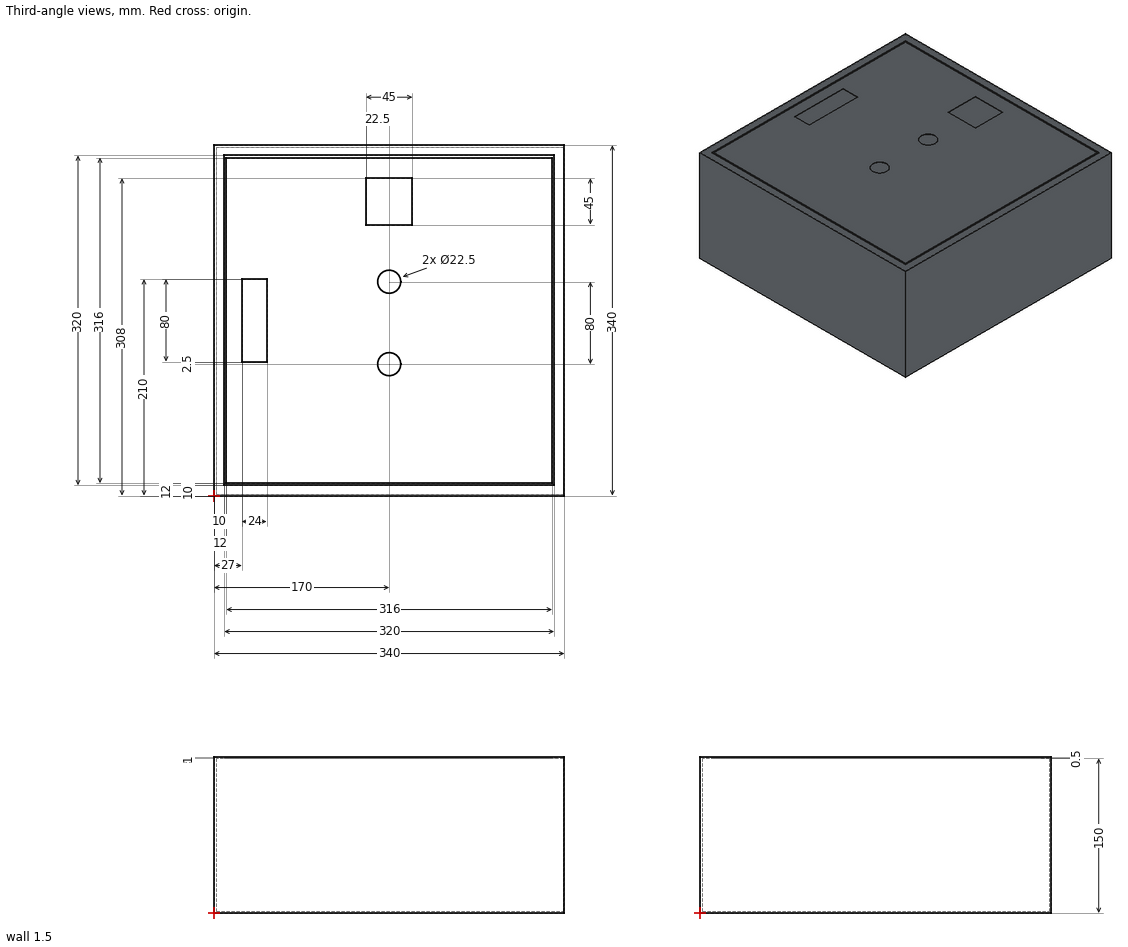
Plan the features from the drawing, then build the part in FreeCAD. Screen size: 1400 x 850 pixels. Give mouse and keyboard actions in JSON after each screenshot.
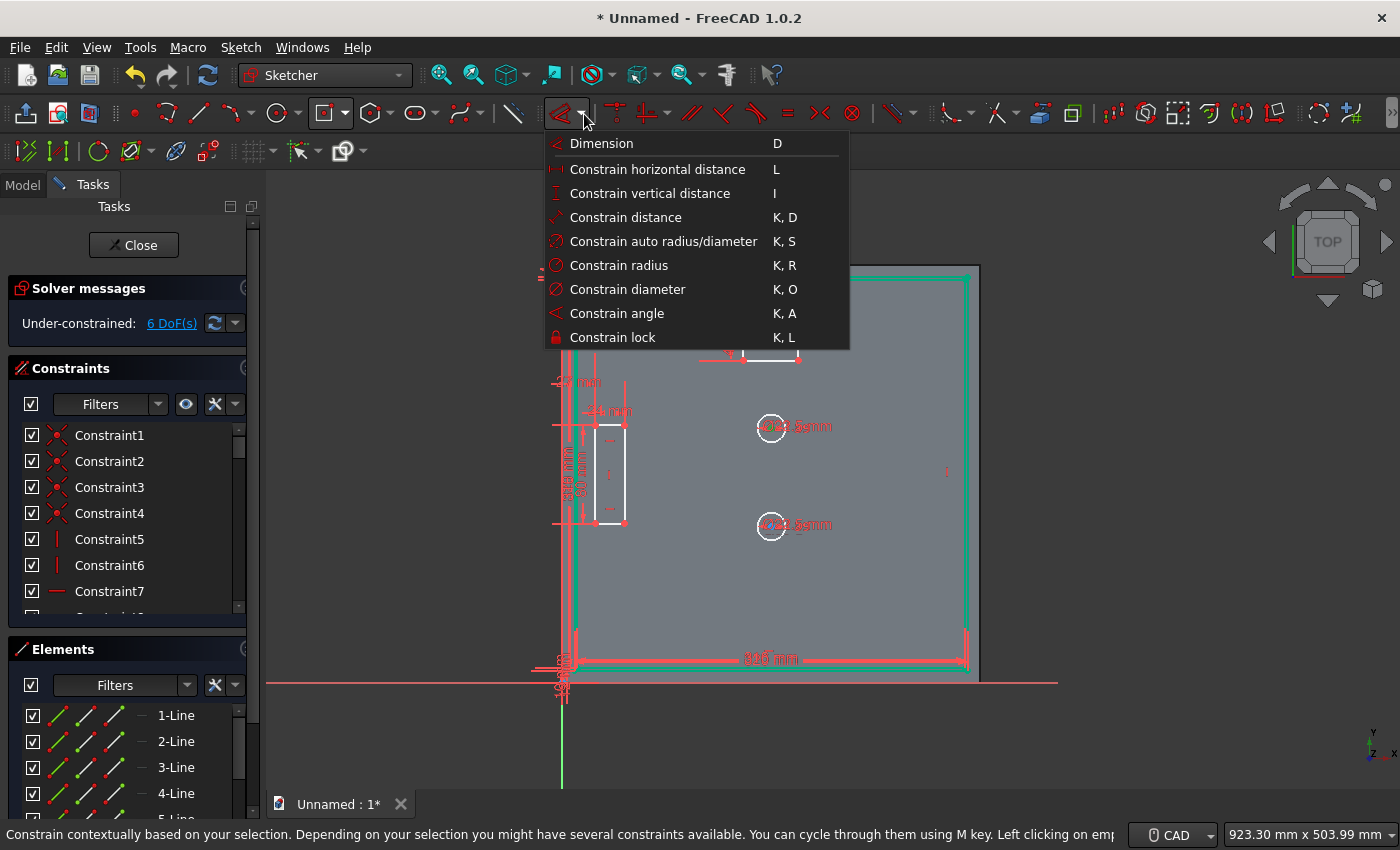
{"action": "left_click", "coordinate": [697, 169]}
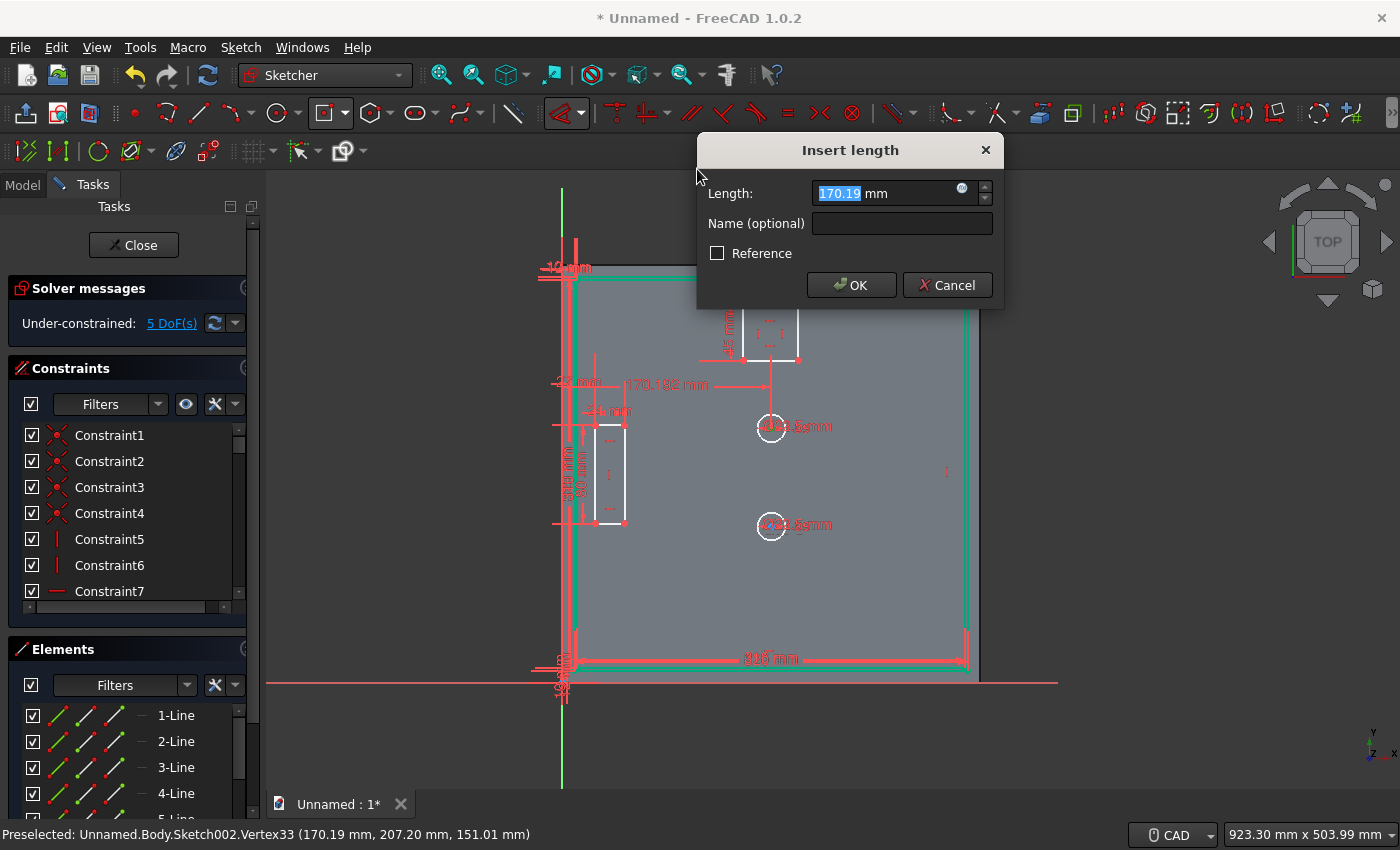
{"action": "type", "text": "170"}
{"action": "key", "text": "Return"}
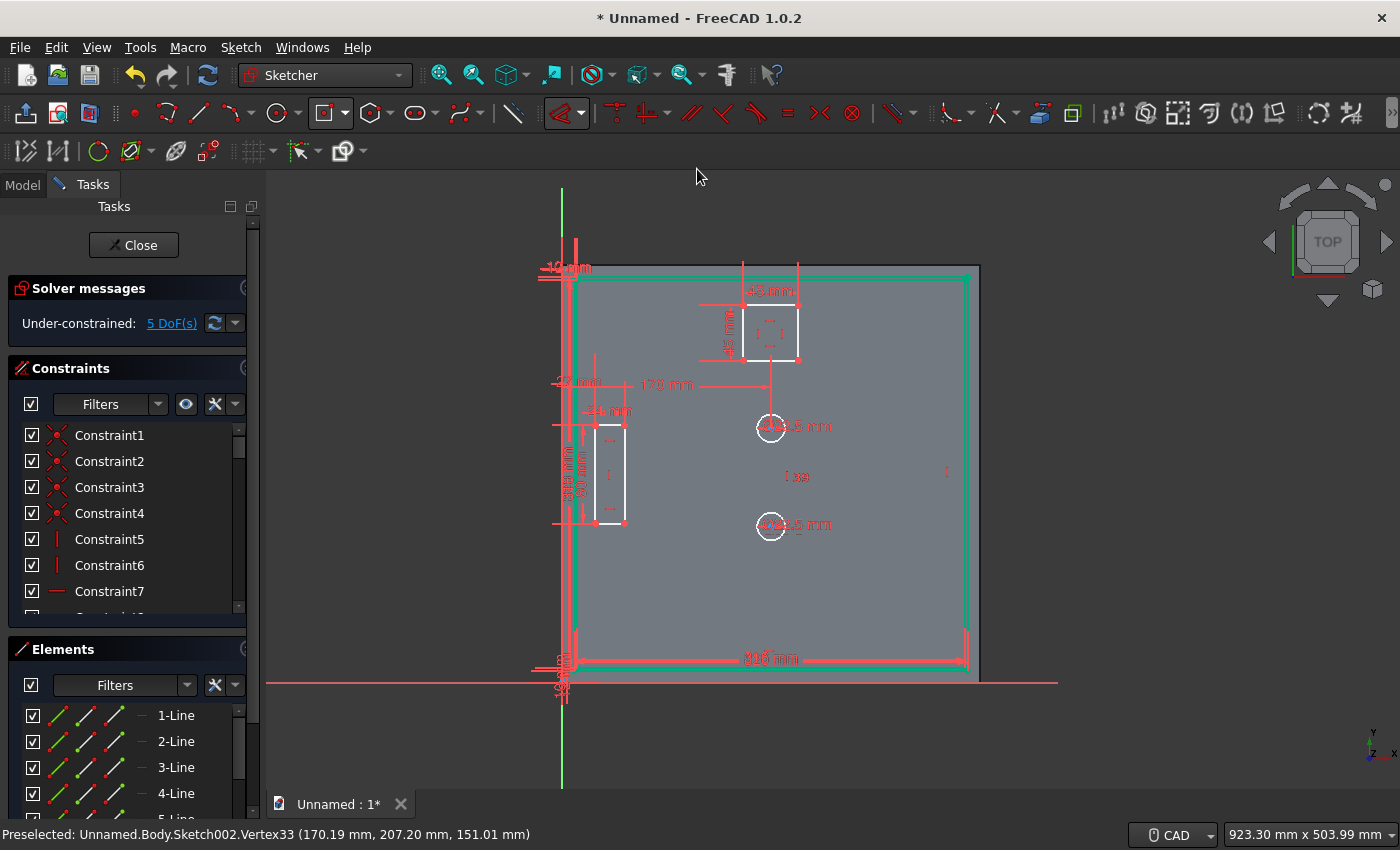
{"action": "left_click", "coordinate": [771, 428]}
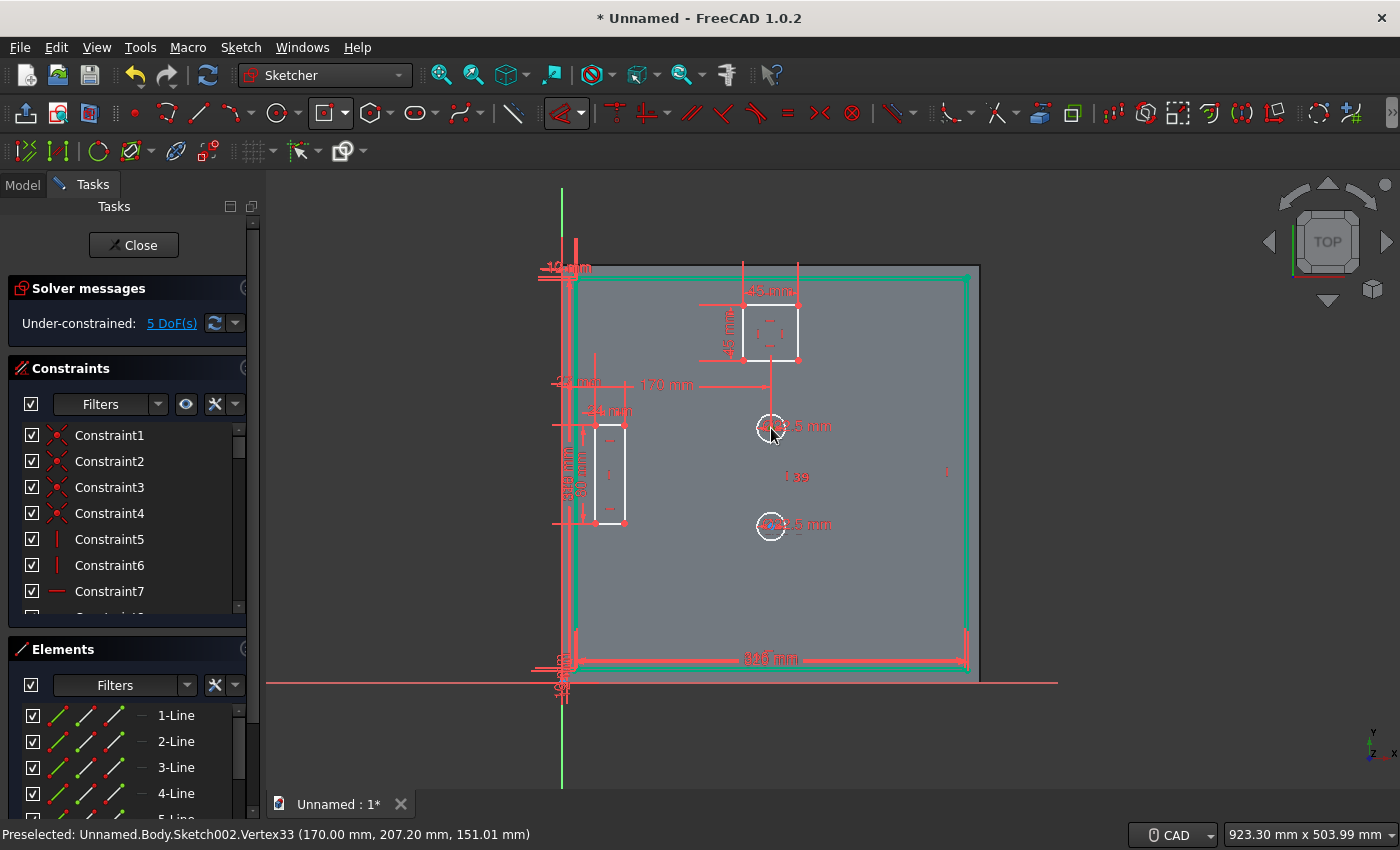
{"action": "left_click", "coordinate": [771, 527]}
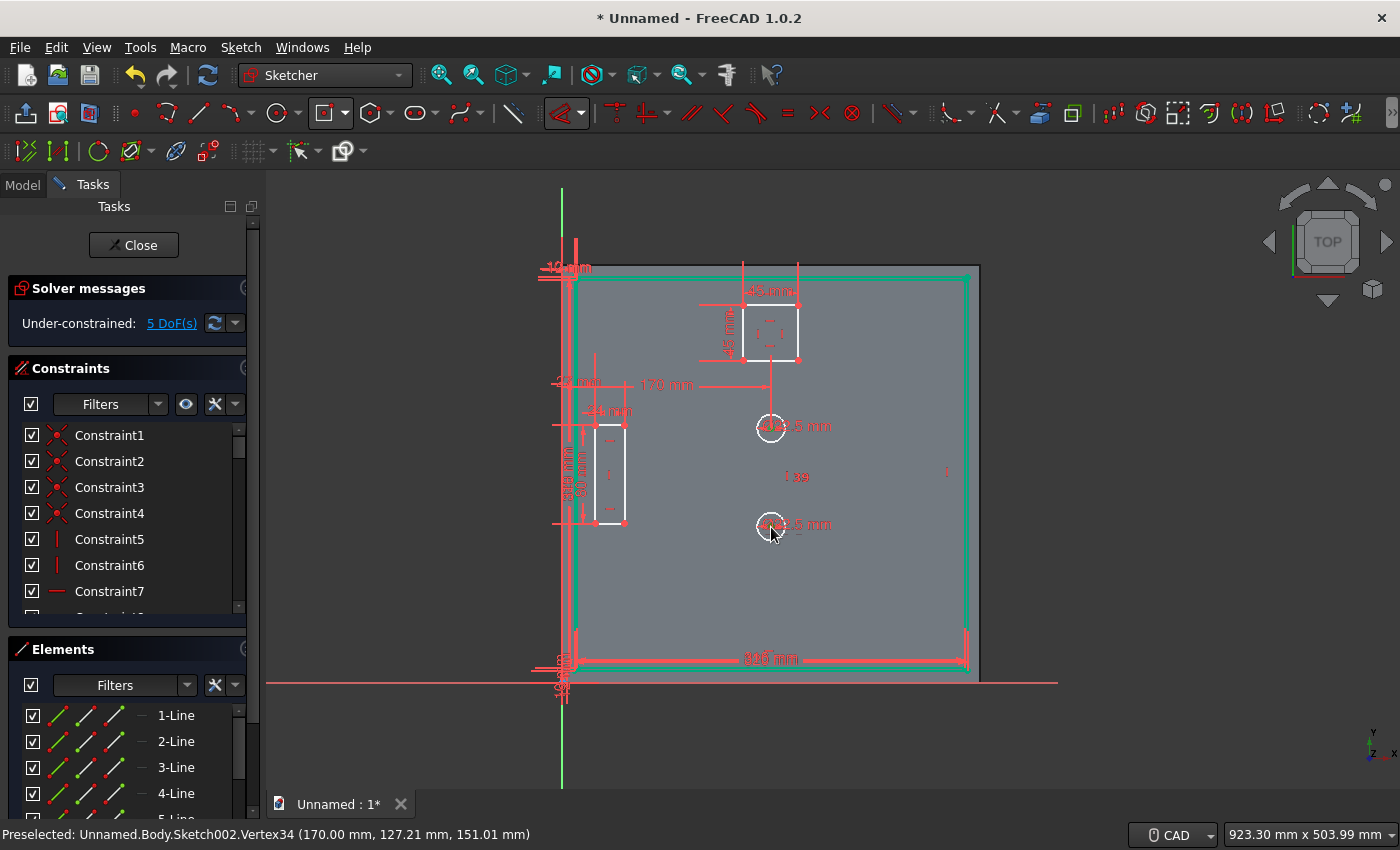
{"action": "key", "text": "i"}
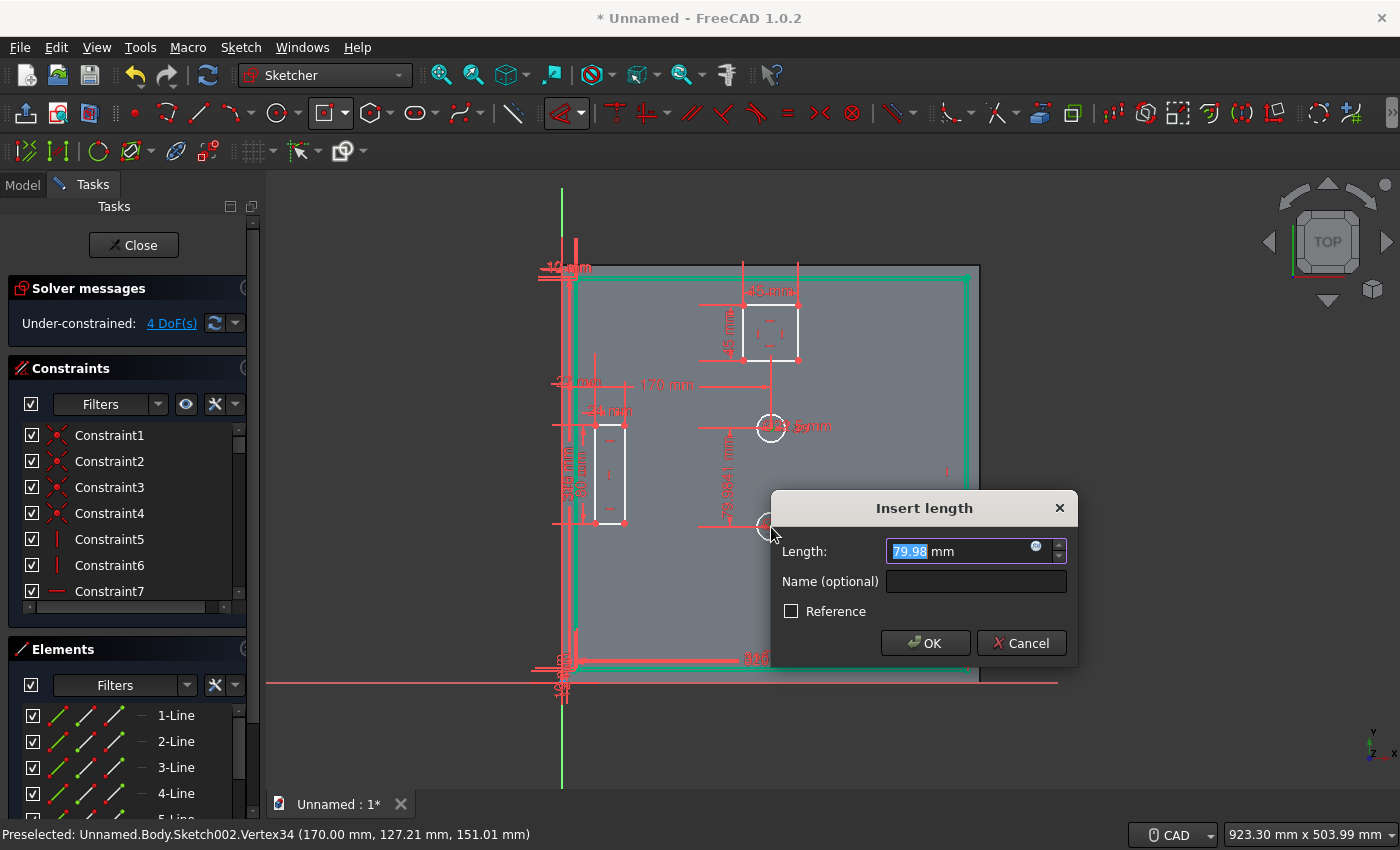
{"action": "type", "text": "80"}
{"action": "key", "text": "Return"}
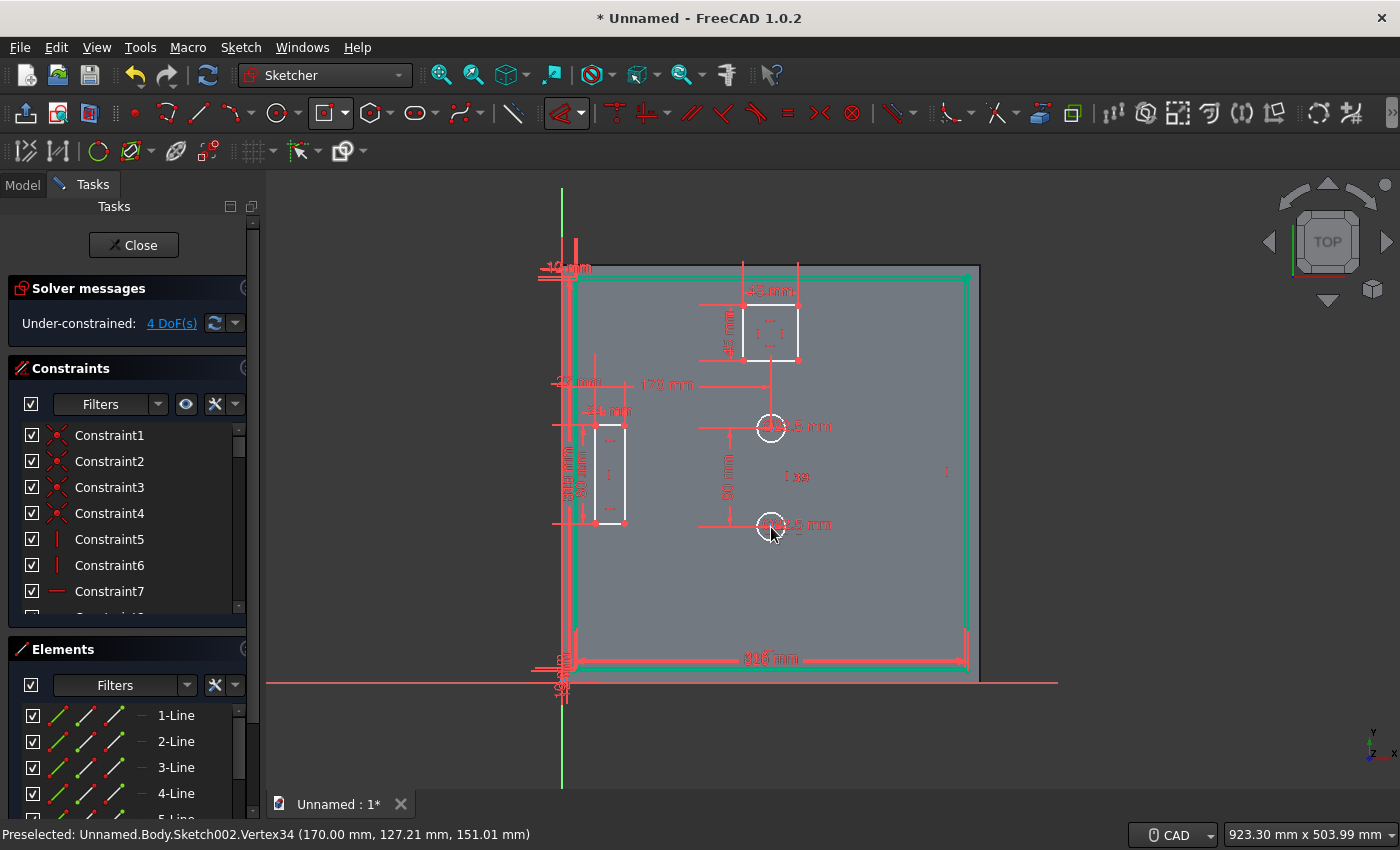
{"action": "left_click", "coordinate": [595, 425]}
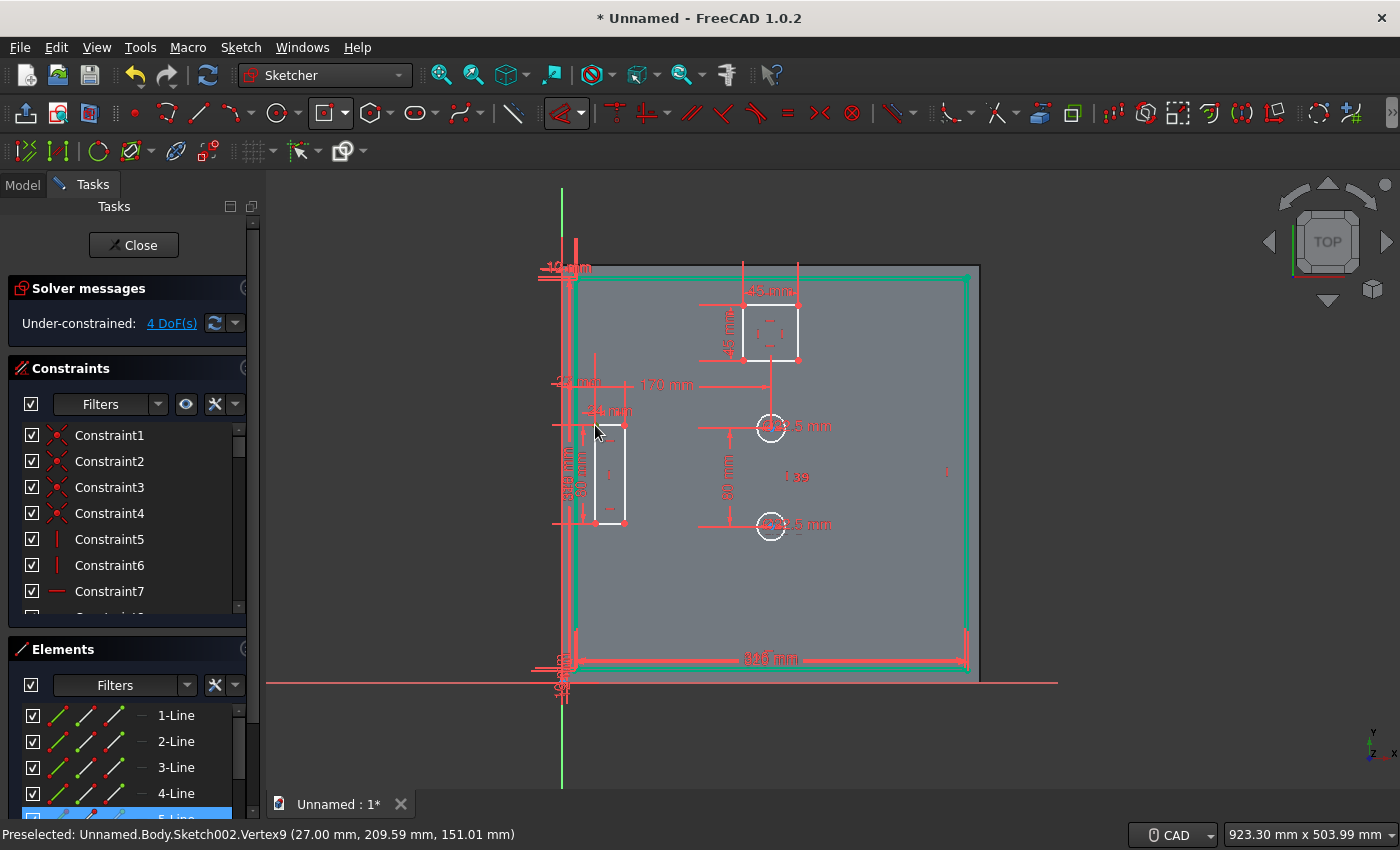
{"action": "key", "text": "i"}